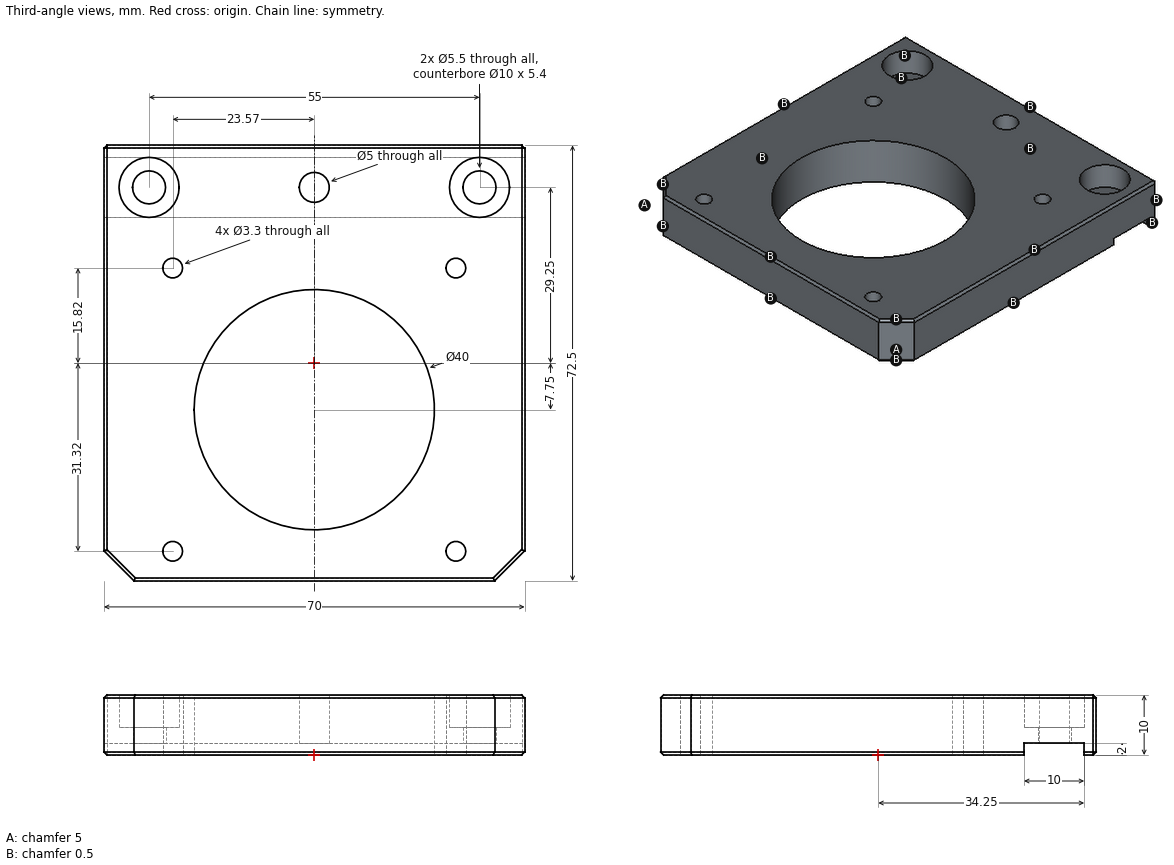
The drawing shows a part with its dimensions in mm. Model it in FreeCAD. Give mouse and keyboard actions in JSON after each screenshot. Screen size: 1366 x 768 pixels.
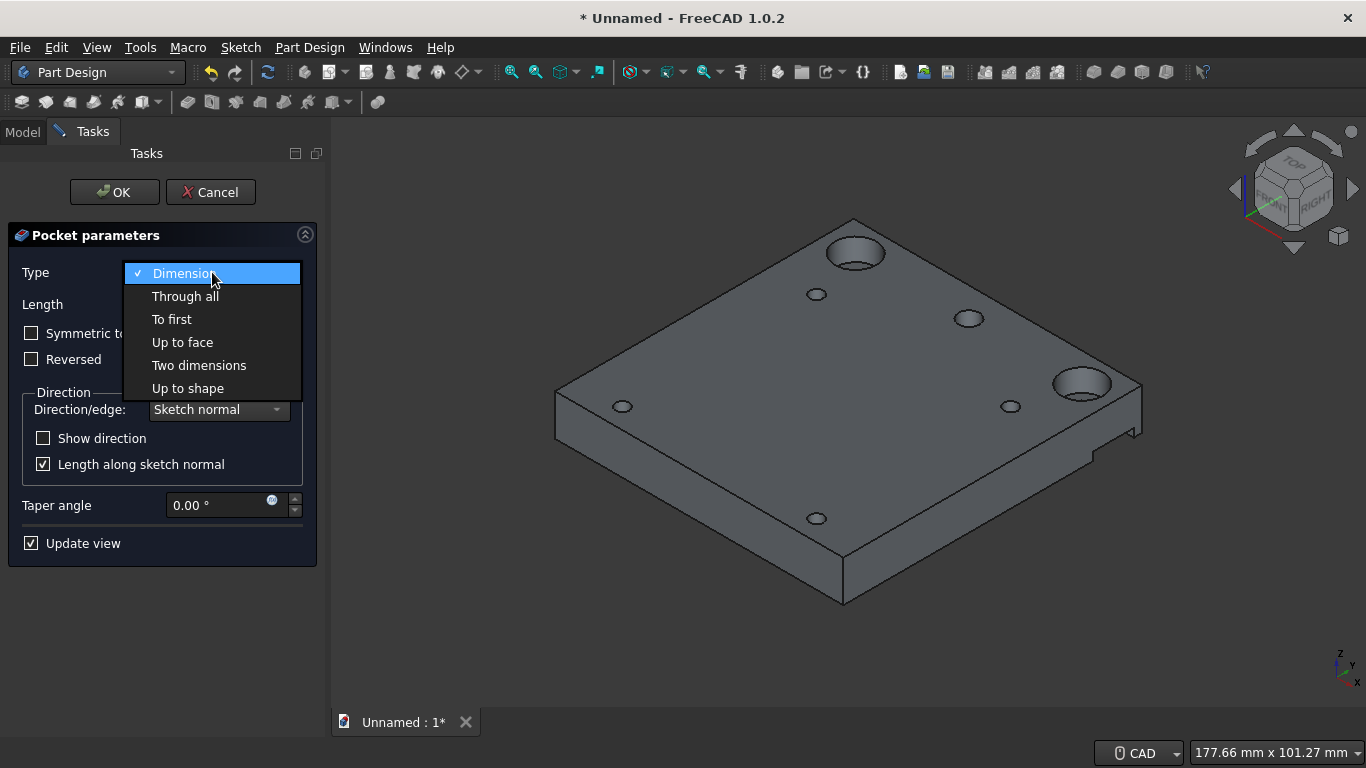
{"action": "left_click", "coordinate": [212, 296]}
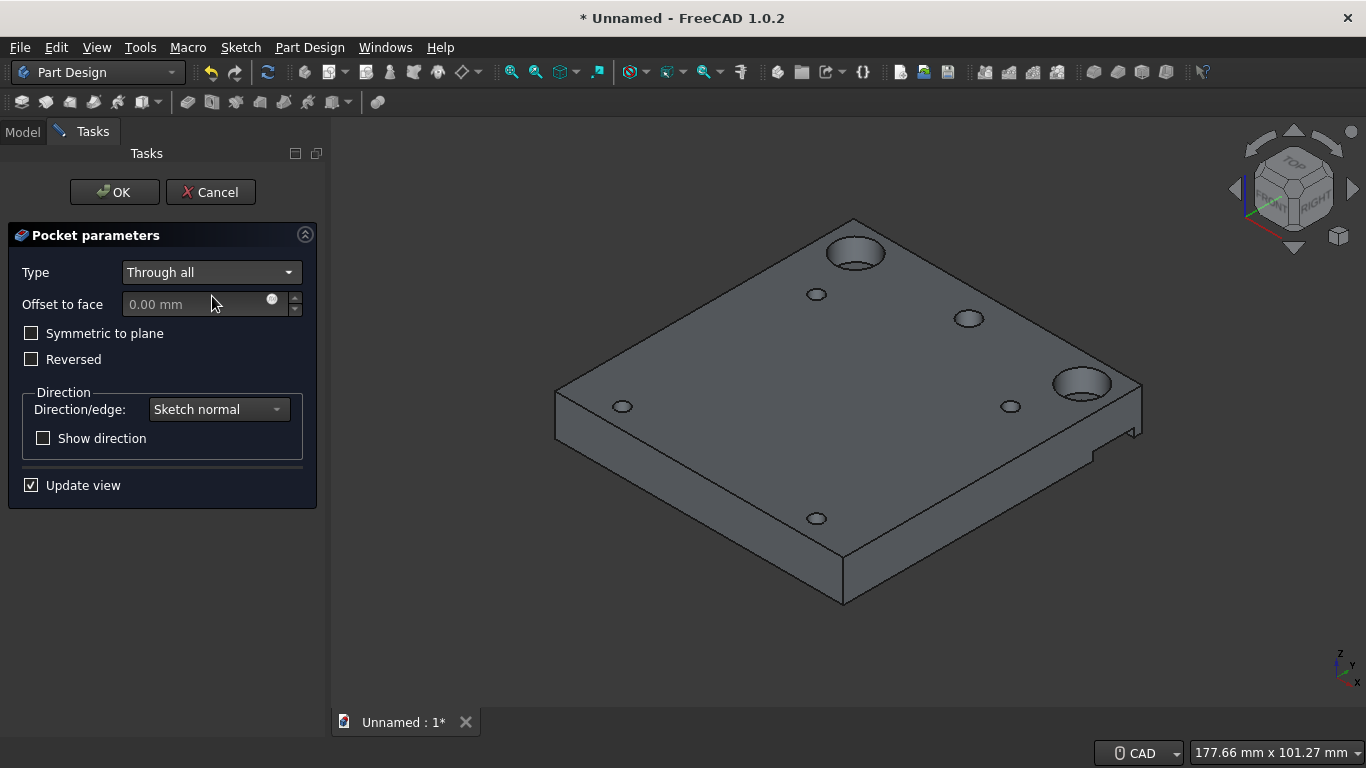
{"action": "left_click", "coordinate": [30, 359]}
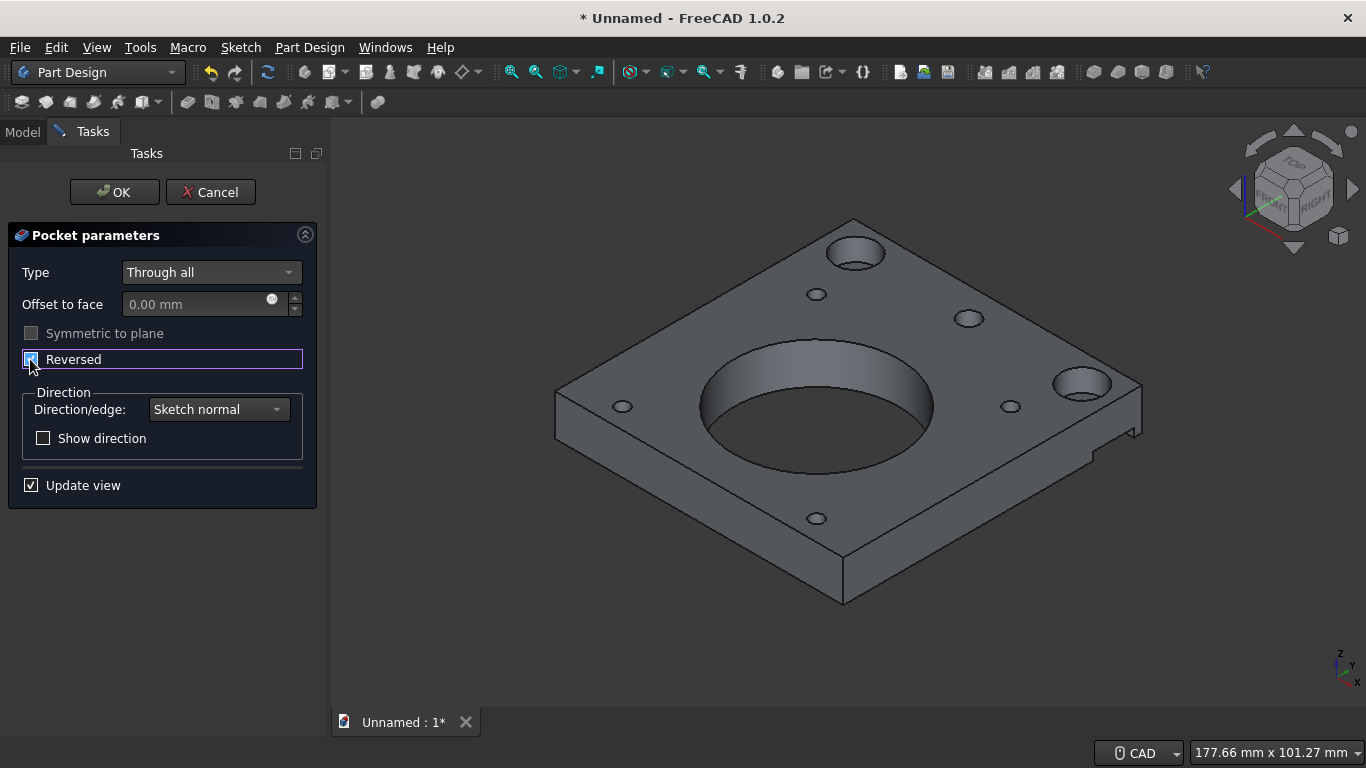
{"action": "left_click", "coordinate": [115, 192]}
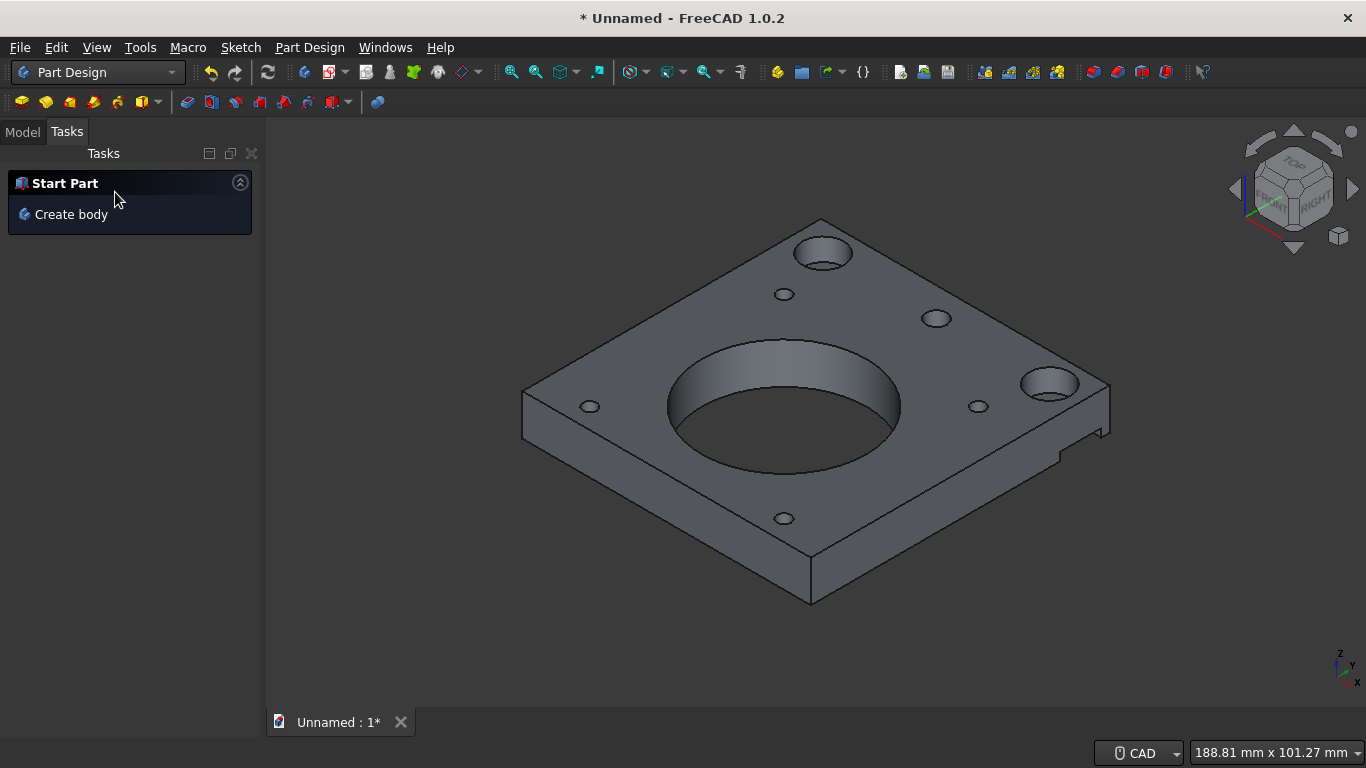
{"action": "left_click", "coordinate": [811, 580]}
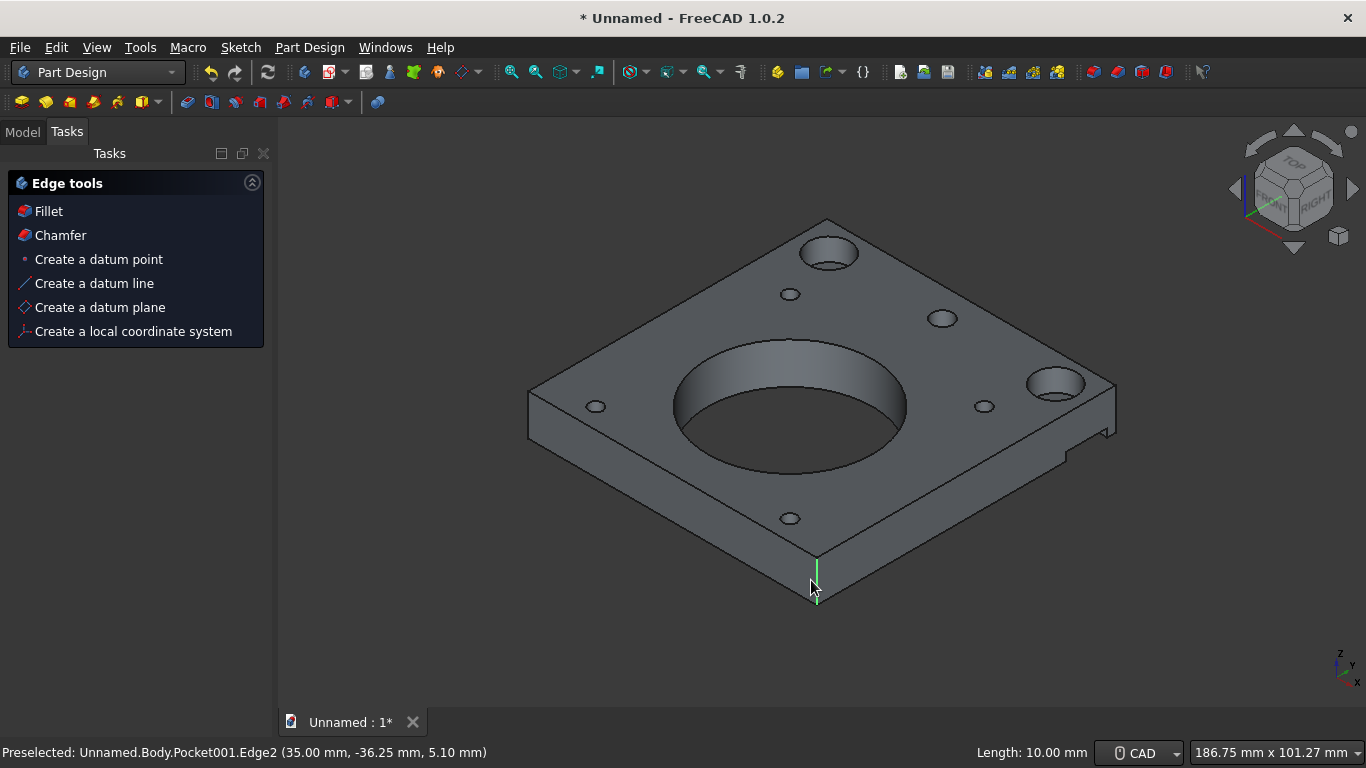
{"action": "key", "text": "2"}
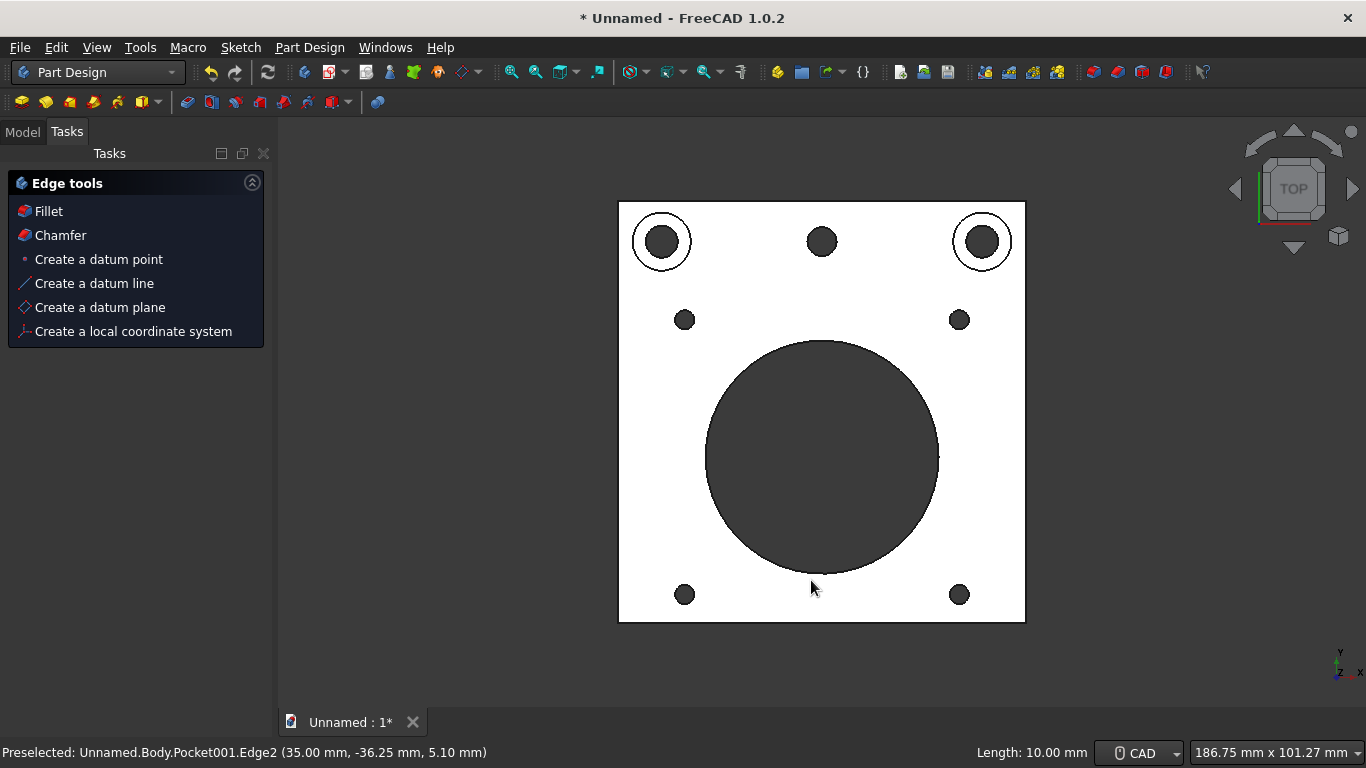
{"action": "key", "text": "0"}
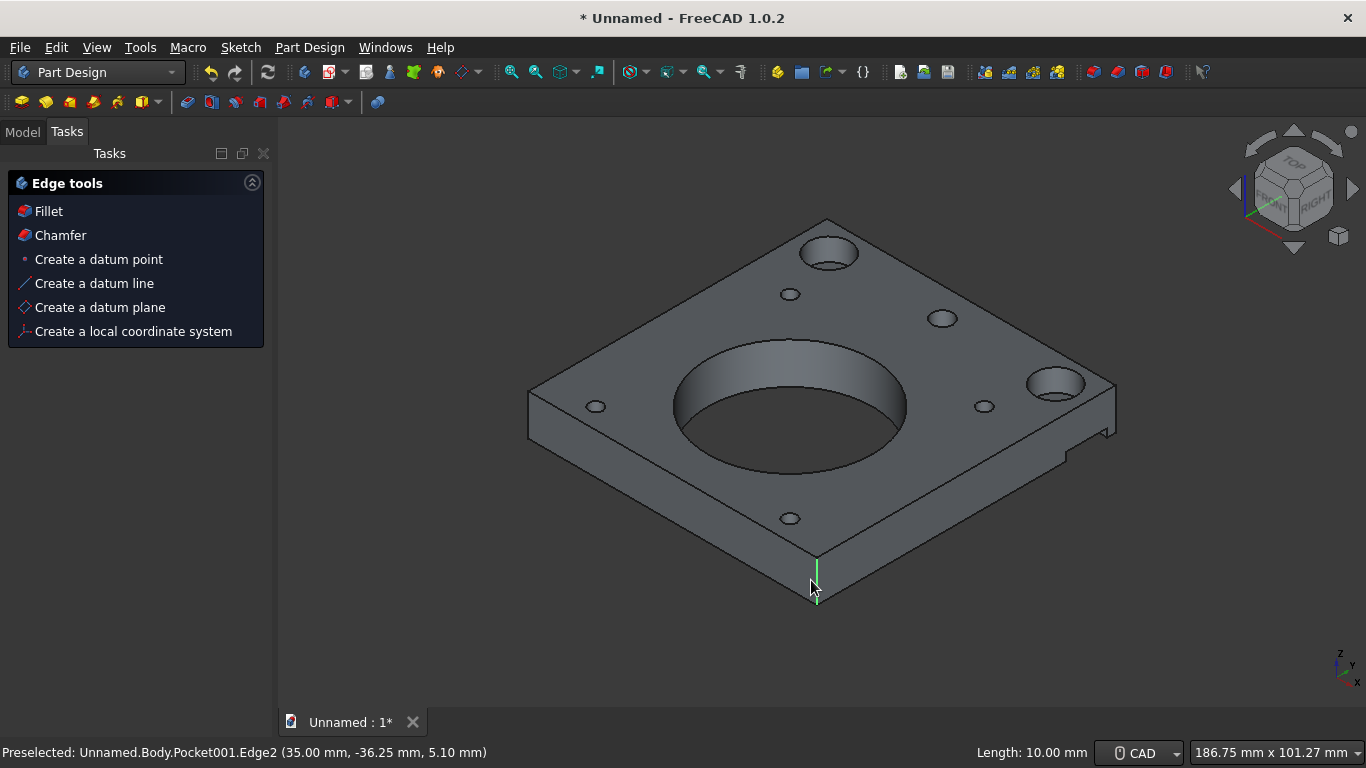
{"action": "key", "text": "1"}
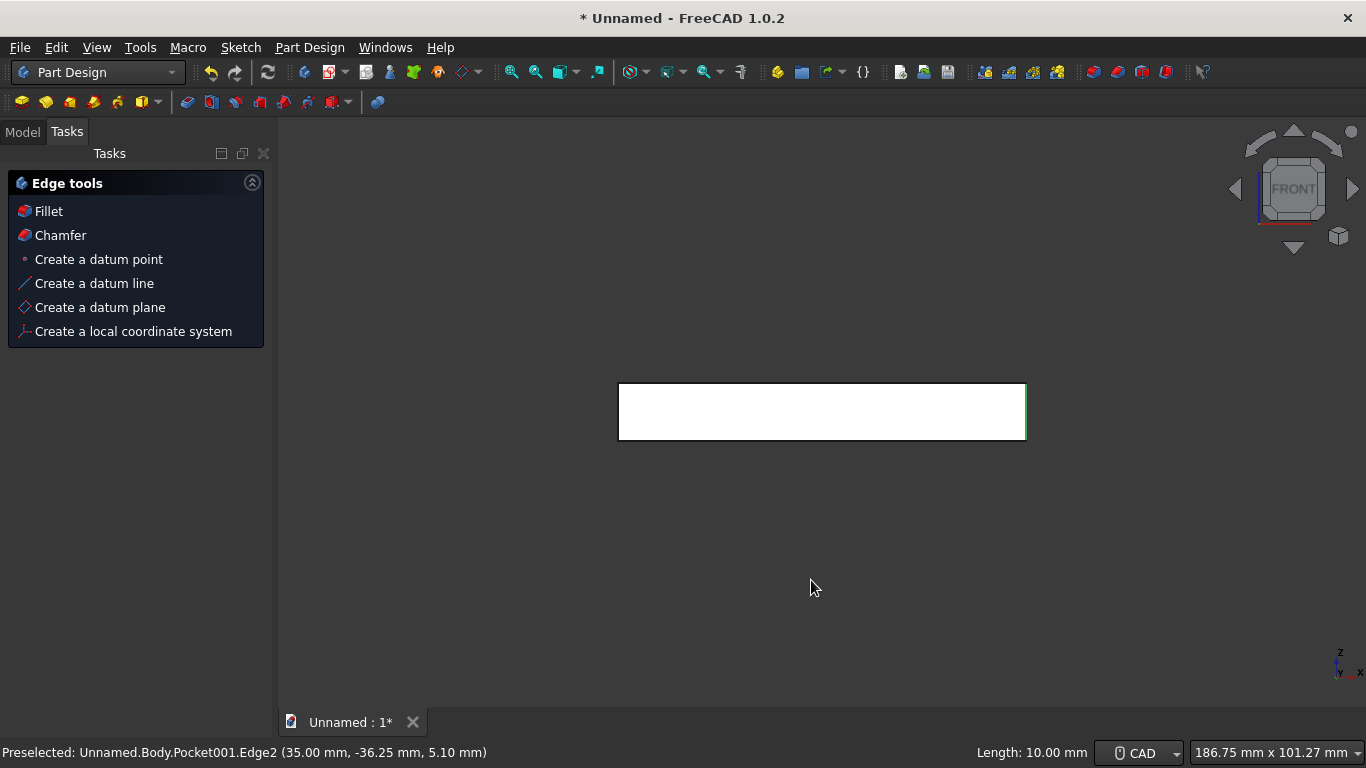
{"action": "left_click", "coordinate": [512, 72]}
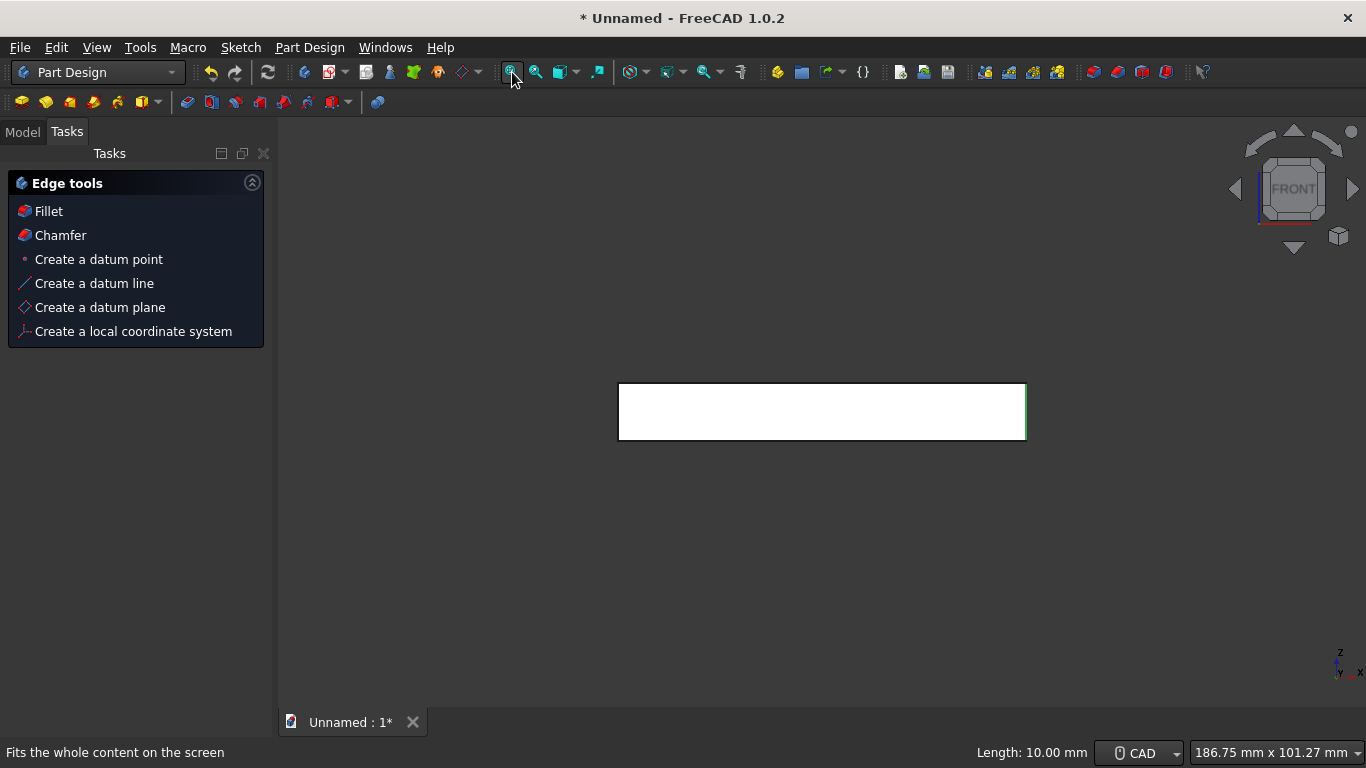
{"action": "left_click", "coordinate": [618, 411], "text": "ctrl"}